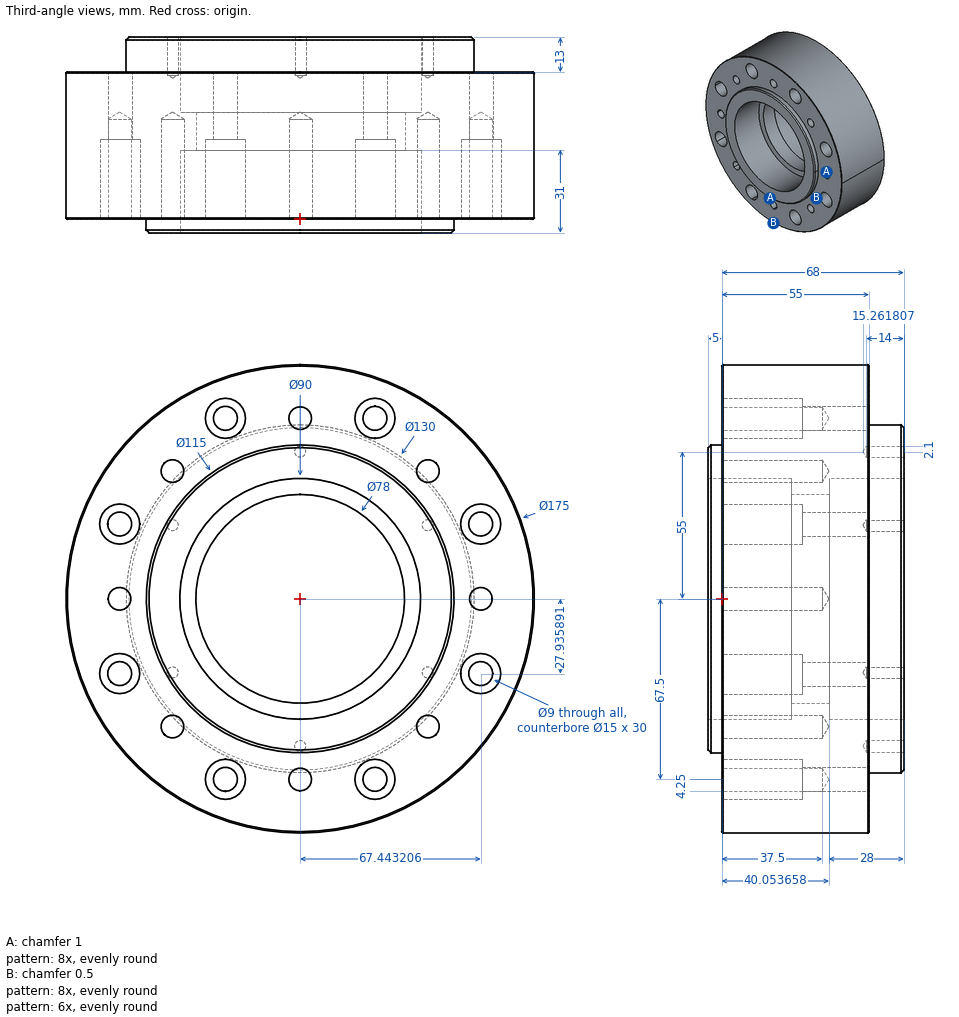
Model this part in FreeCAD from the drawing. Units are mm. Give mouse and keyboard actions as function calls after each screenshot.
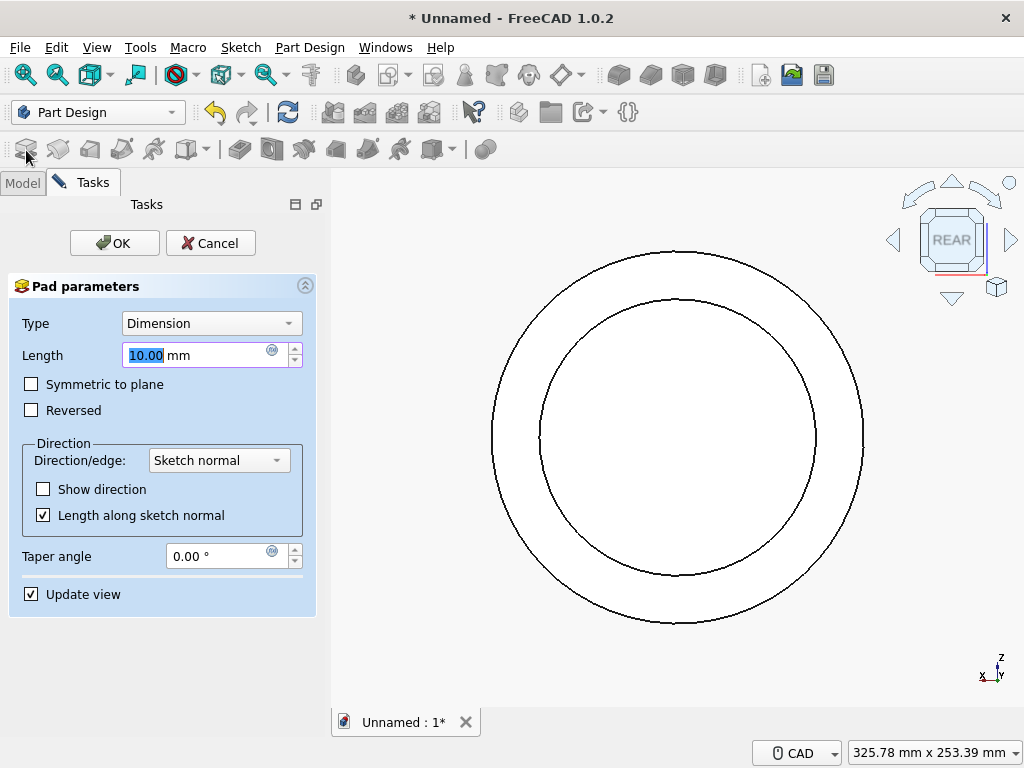
text(13)
key(Tab)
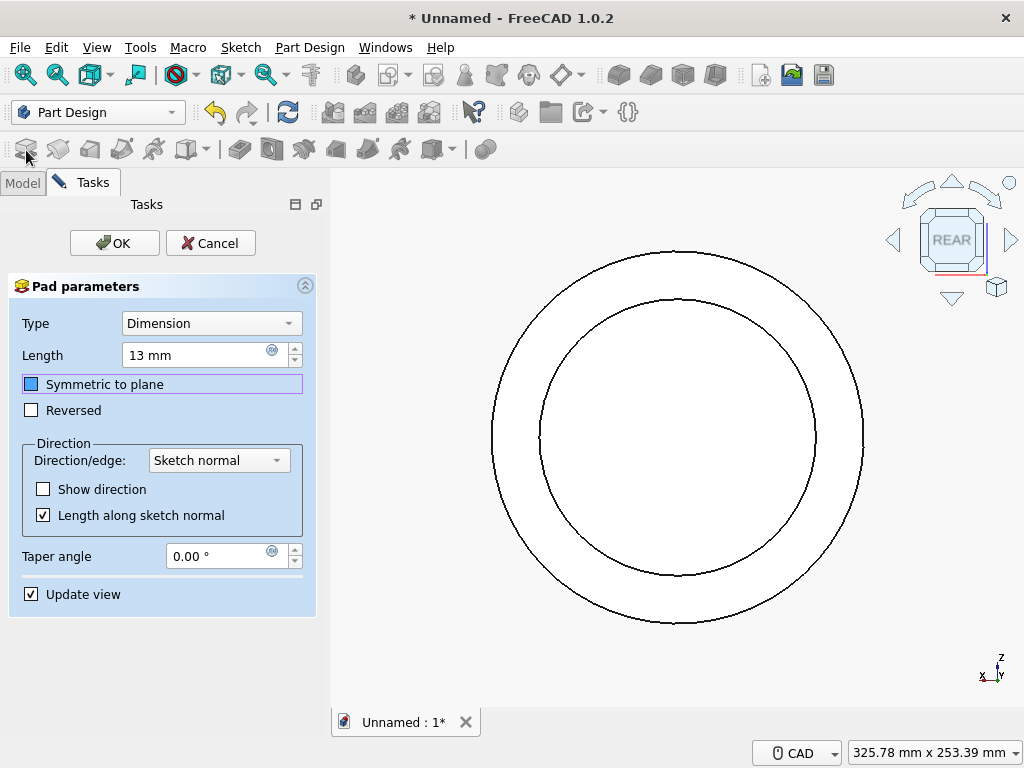
click(115, 243)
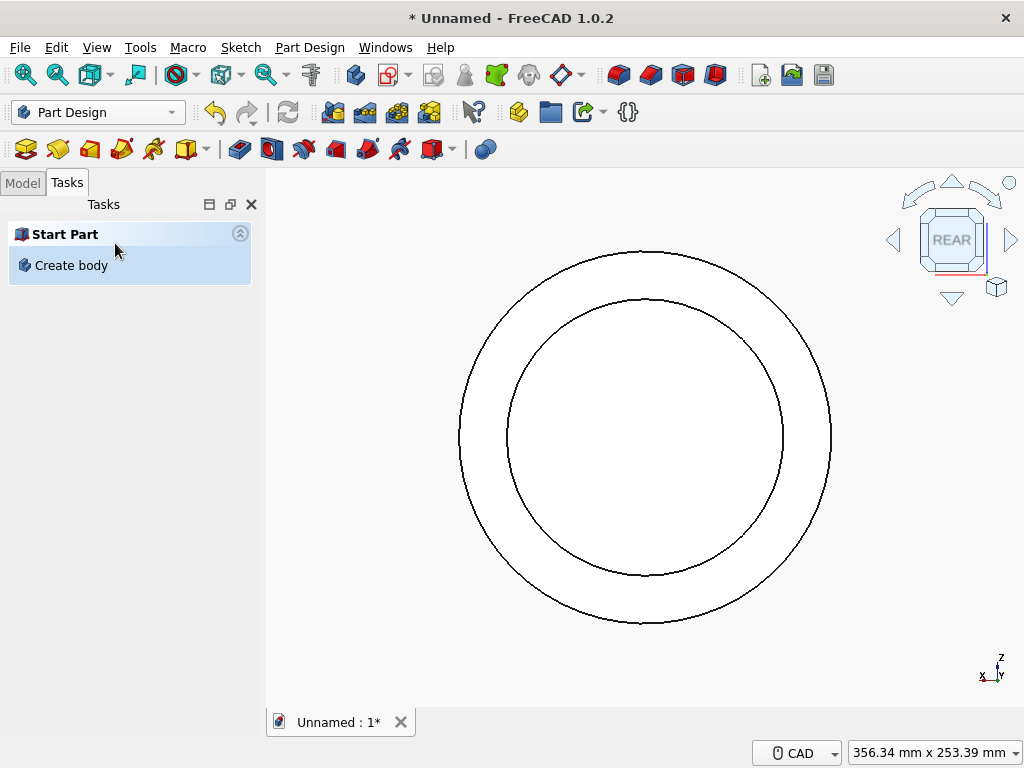
click(388, 76)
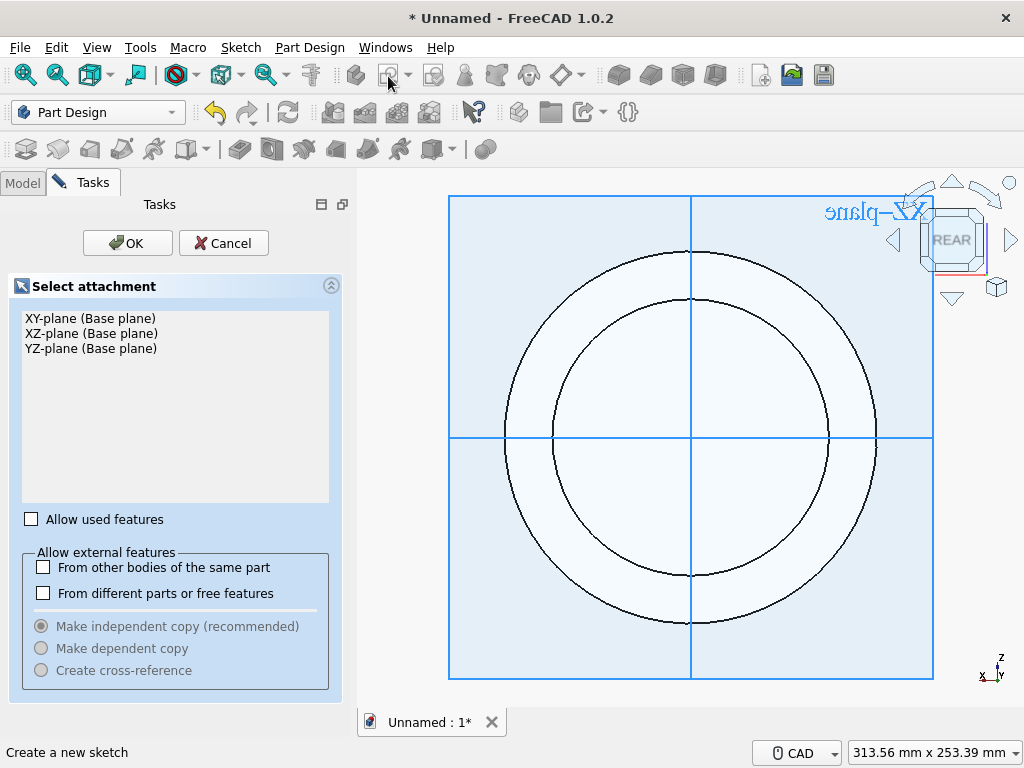
click(82, 334)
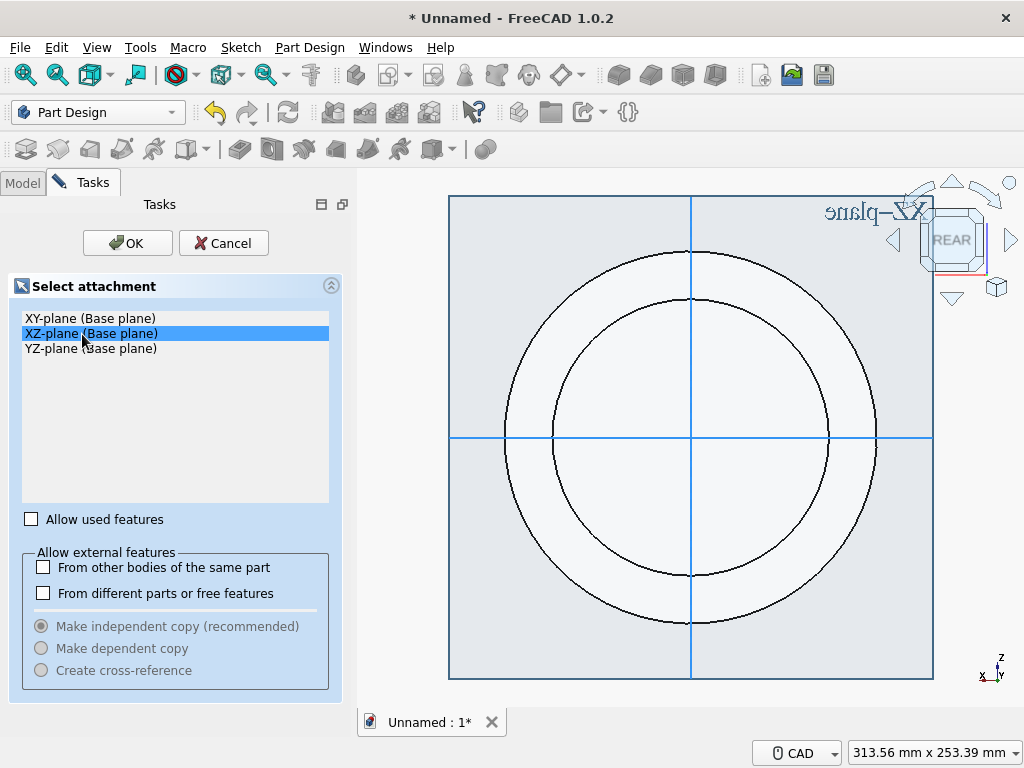
click(128, 243)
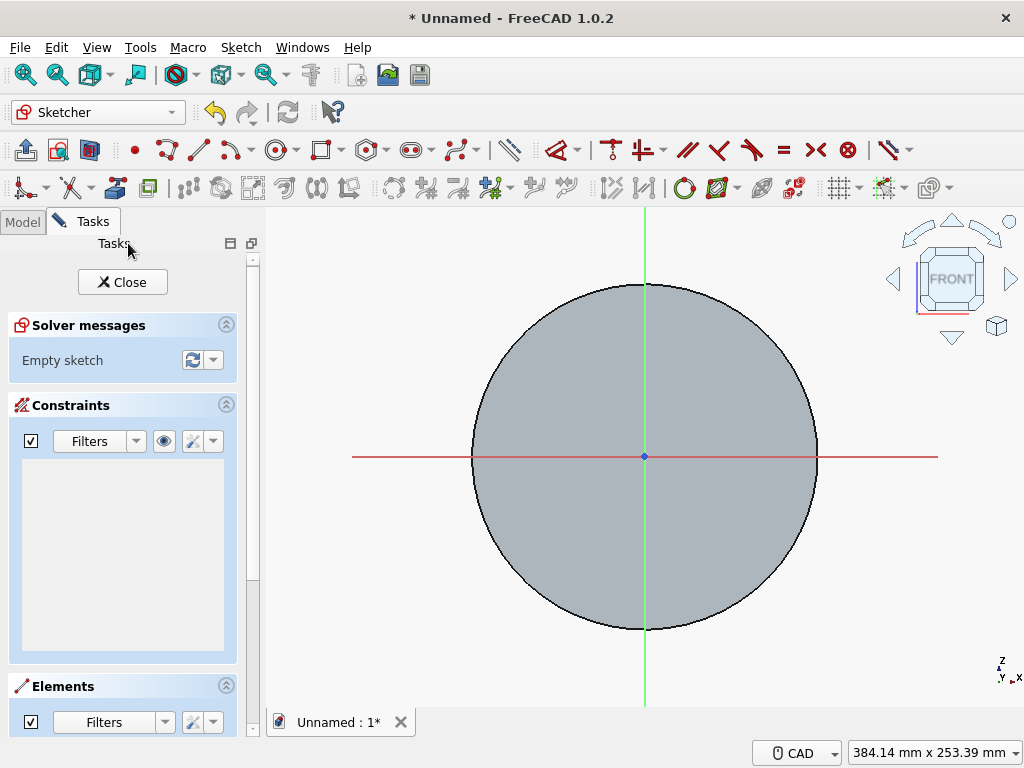
scroll(784, 457, up, 2)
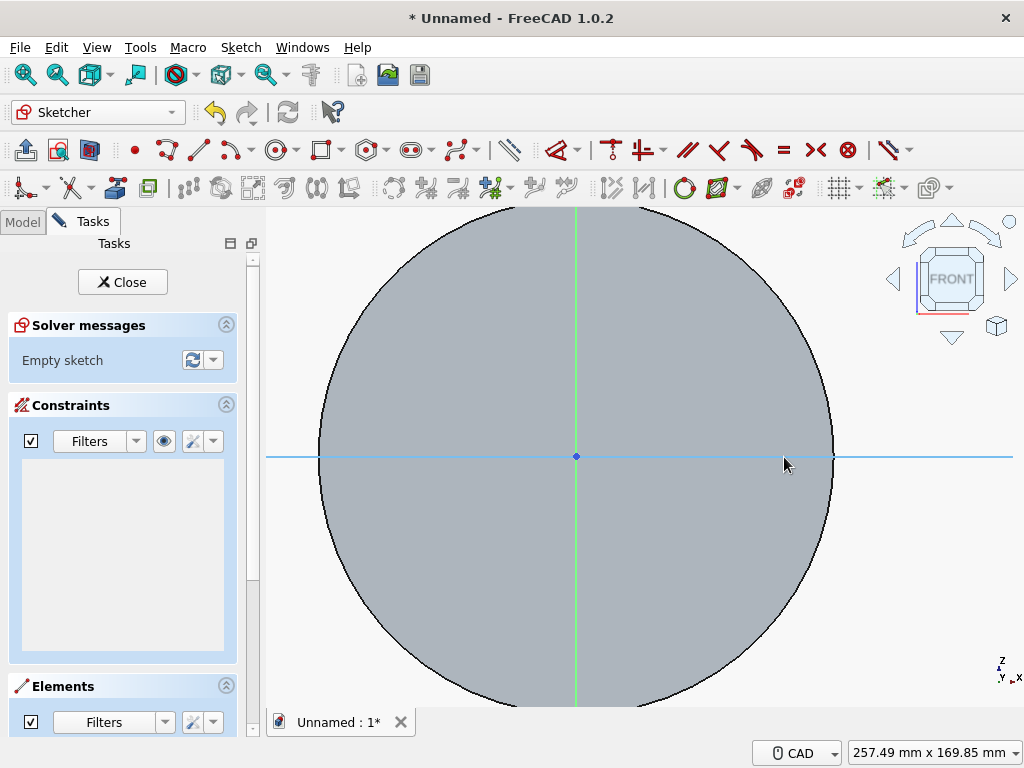
click(276, 150)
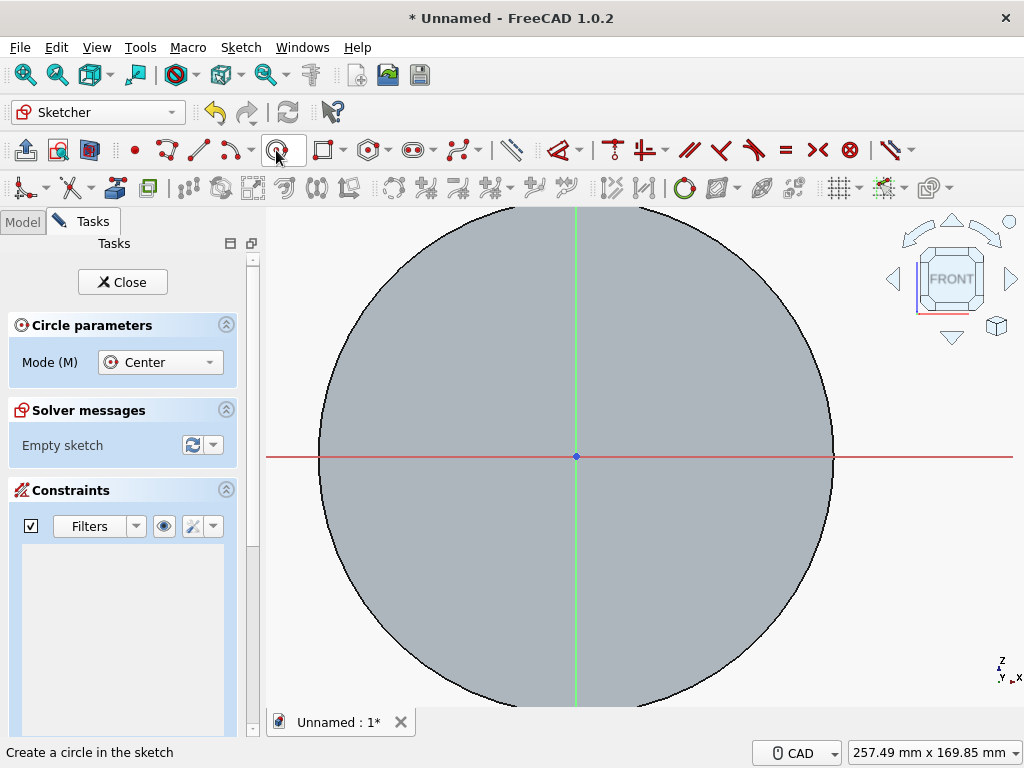
click(576, 457)
click(696, 337)
key(Escape)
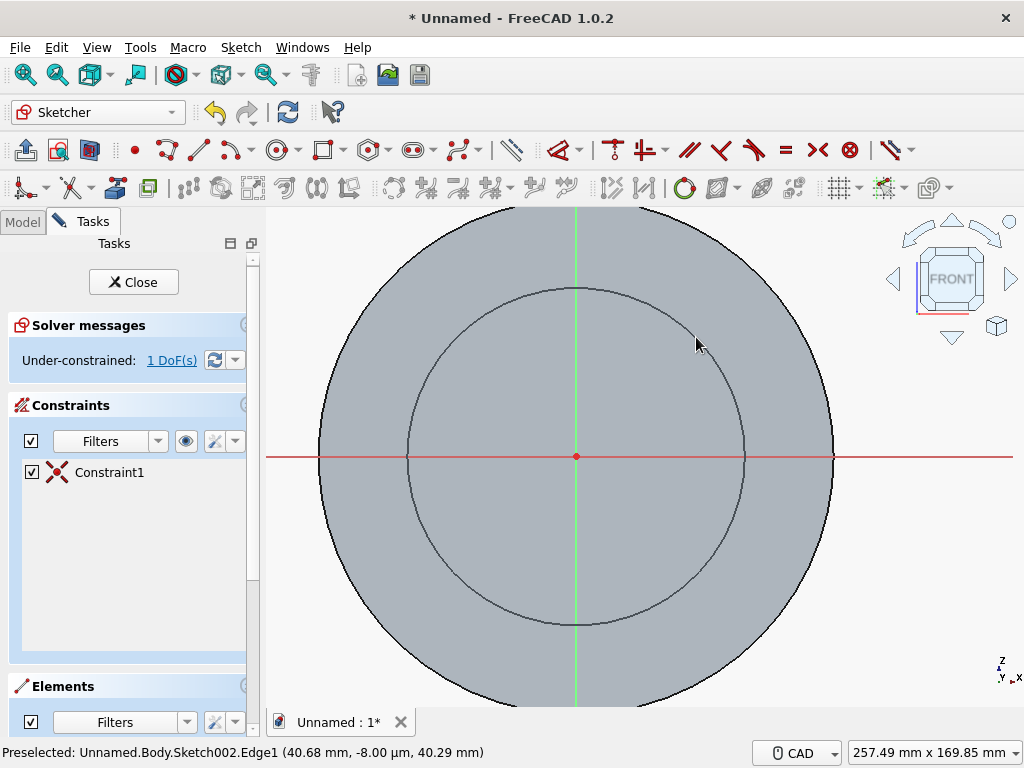
key(d)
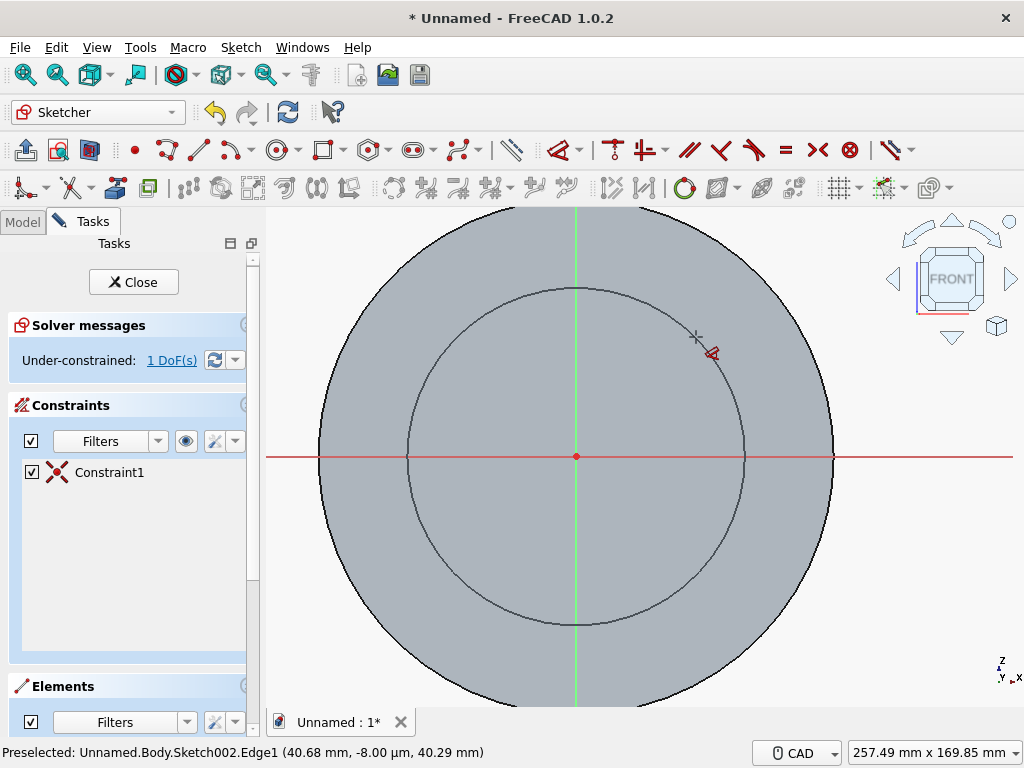
click(695, 337)
click(718, 314)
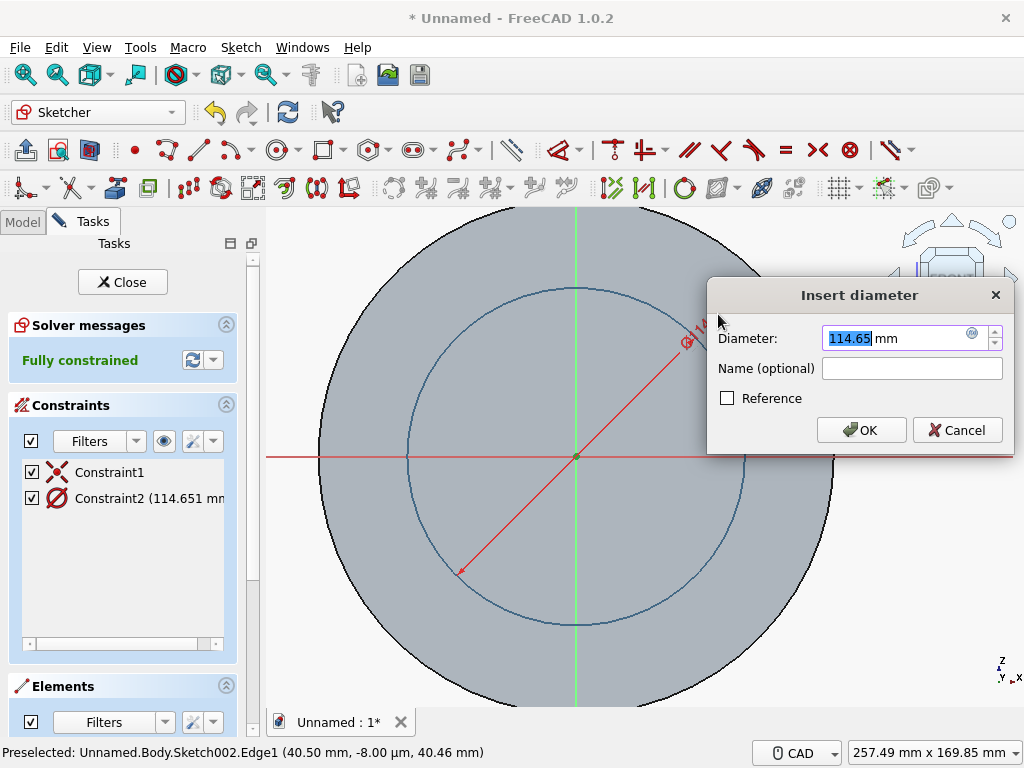
text(115)
key(Return)
key(Escape)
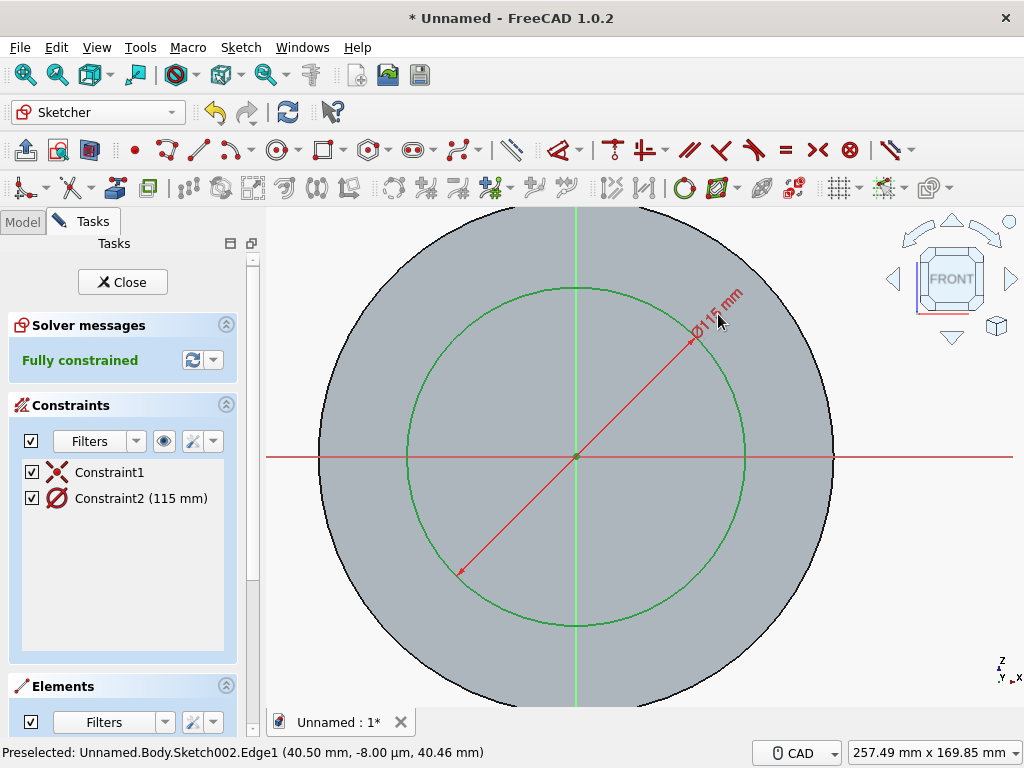
click(123, 282)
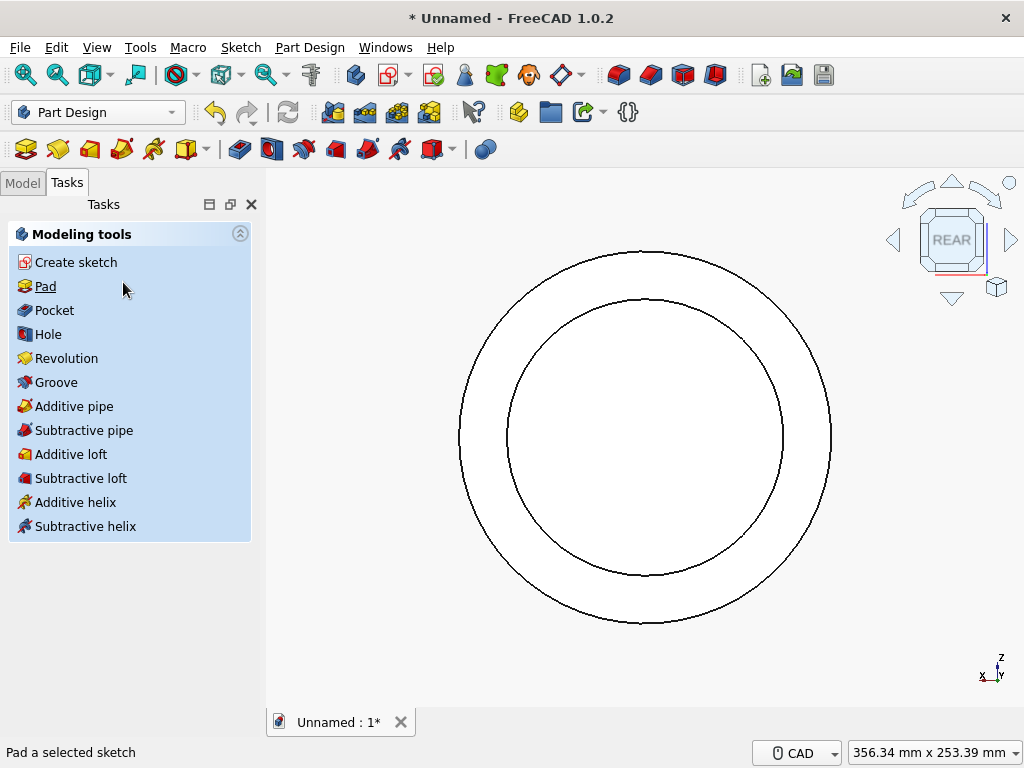
click(26, 150)